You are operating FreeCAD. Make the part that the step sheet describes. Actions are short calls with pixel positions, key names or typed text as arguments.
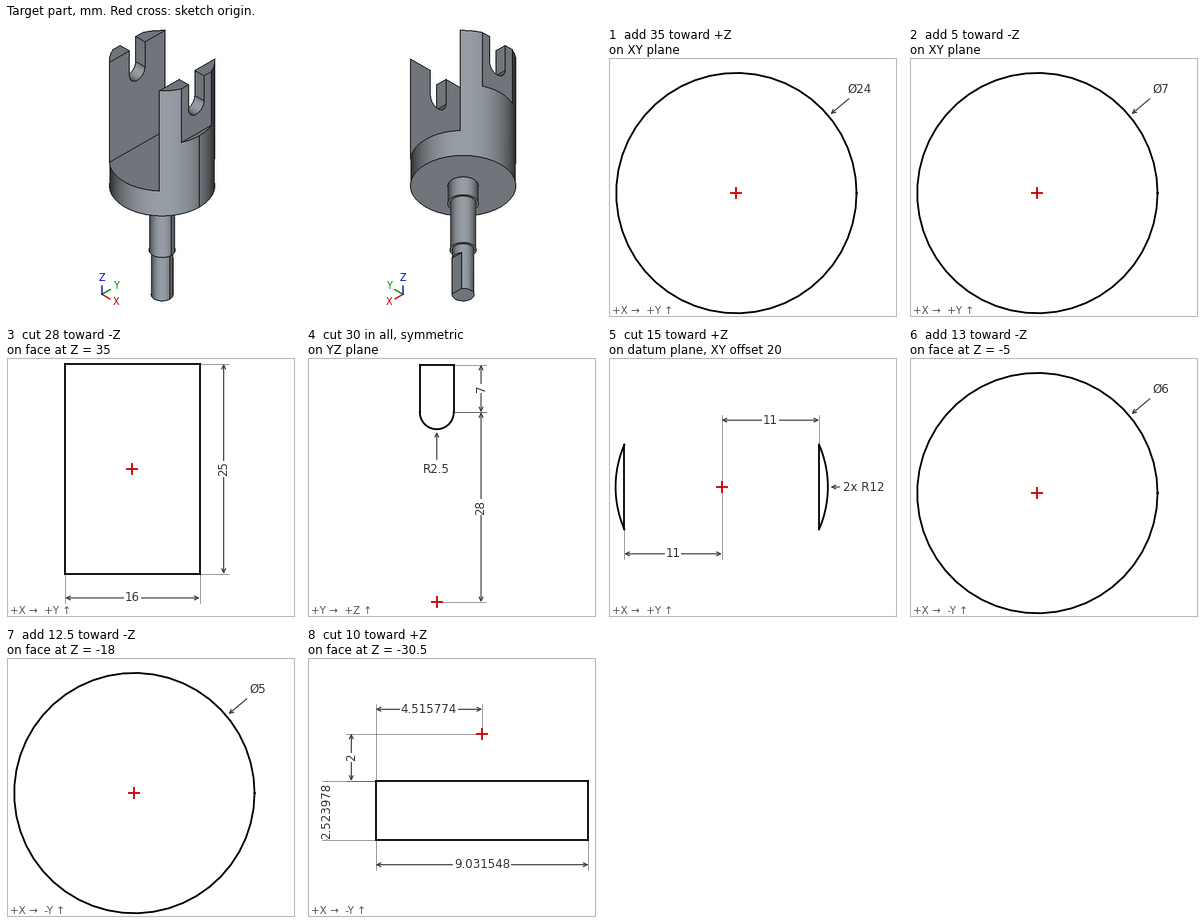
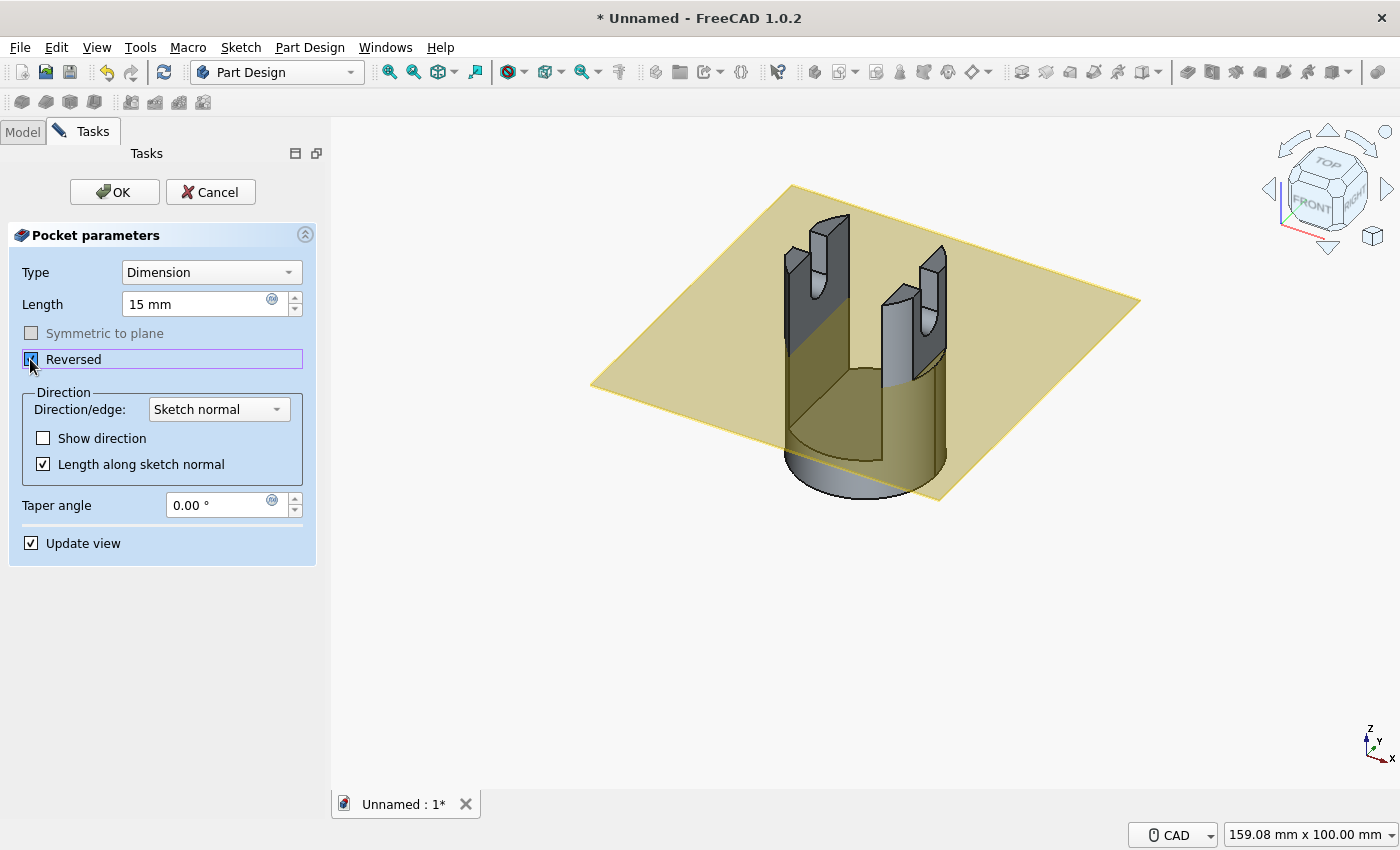
click(115, 192)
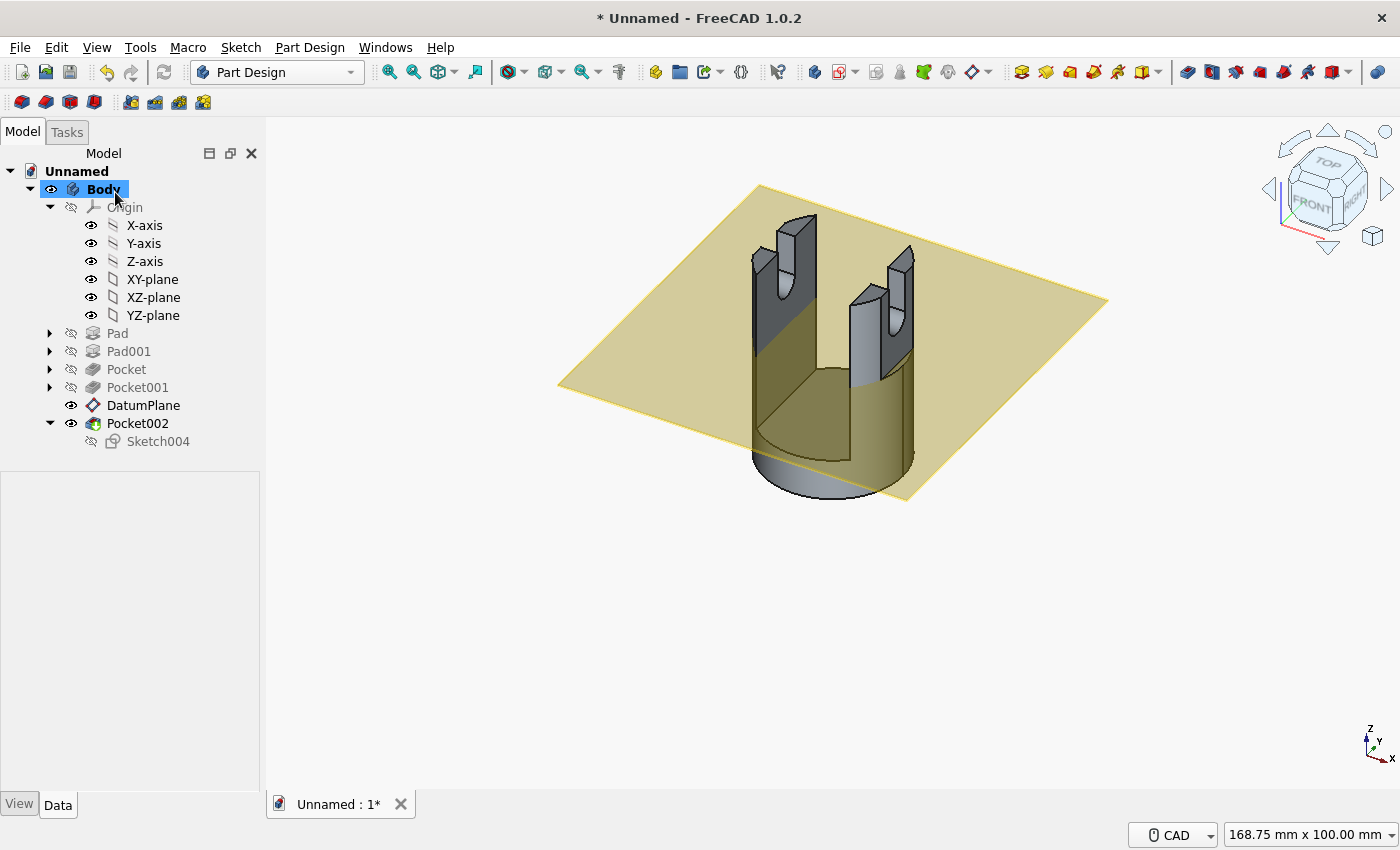
click(116, 405)
key(space)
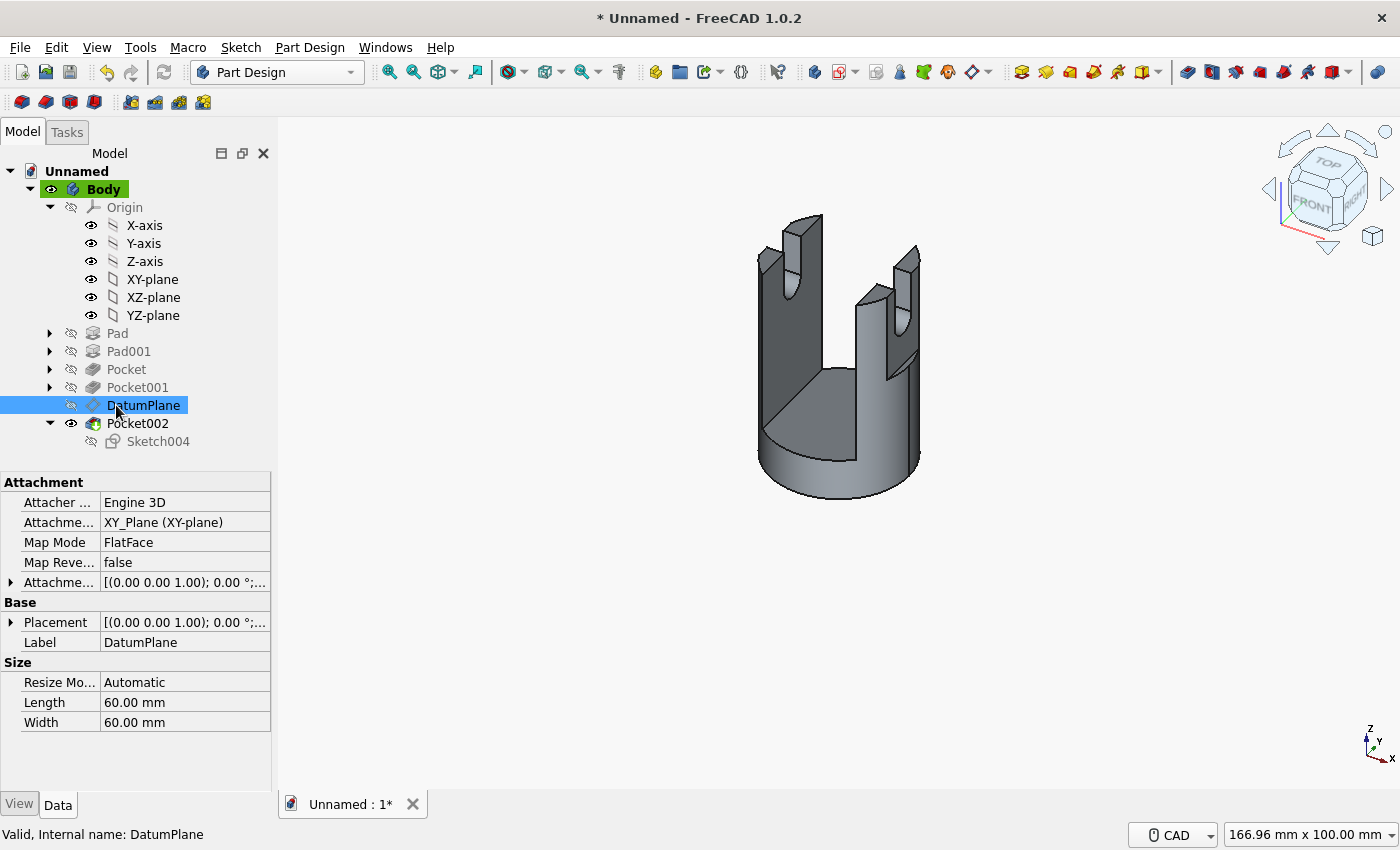
key(5)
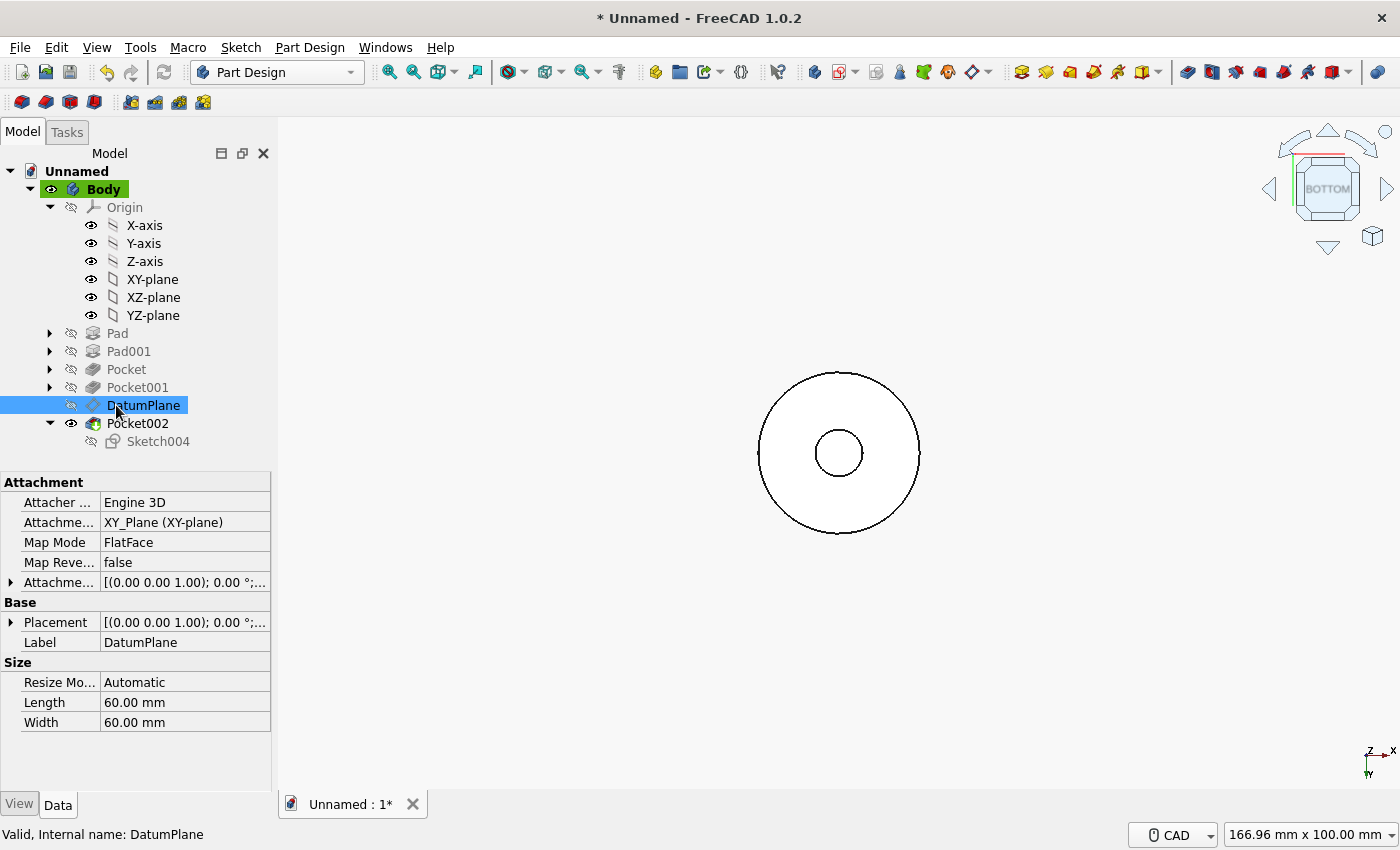
click(390, 72)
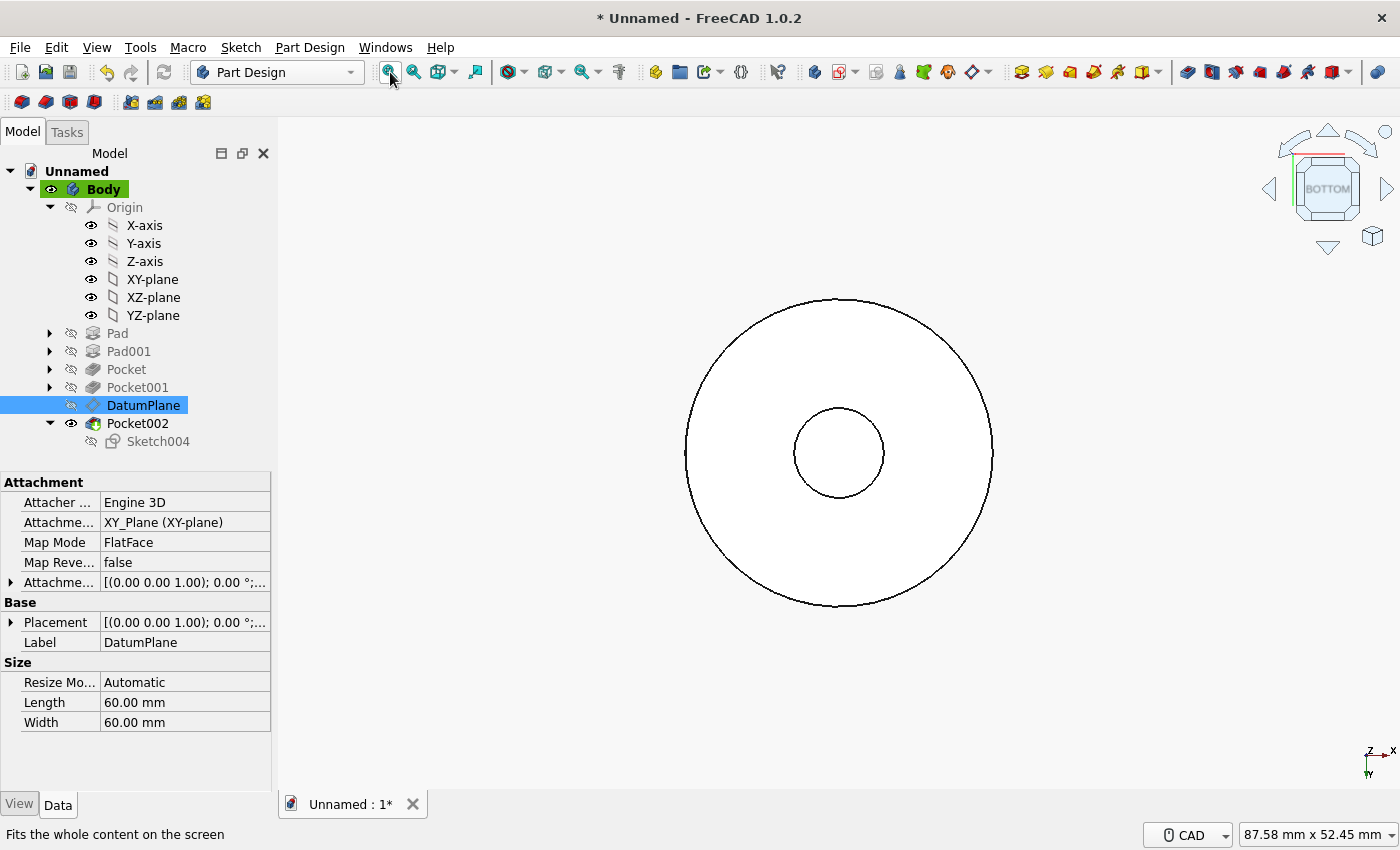
click(839, 452)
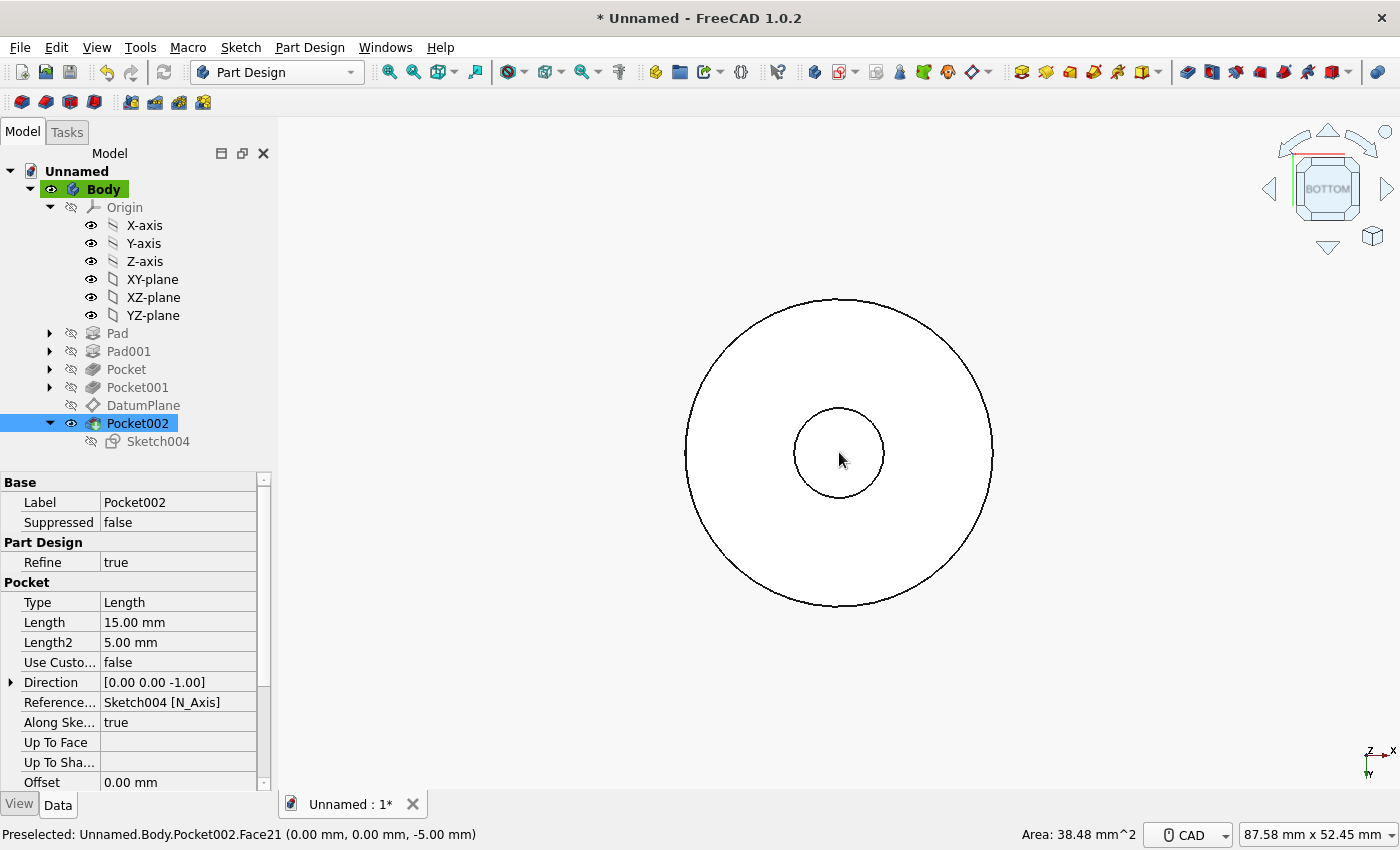
click(840, 72)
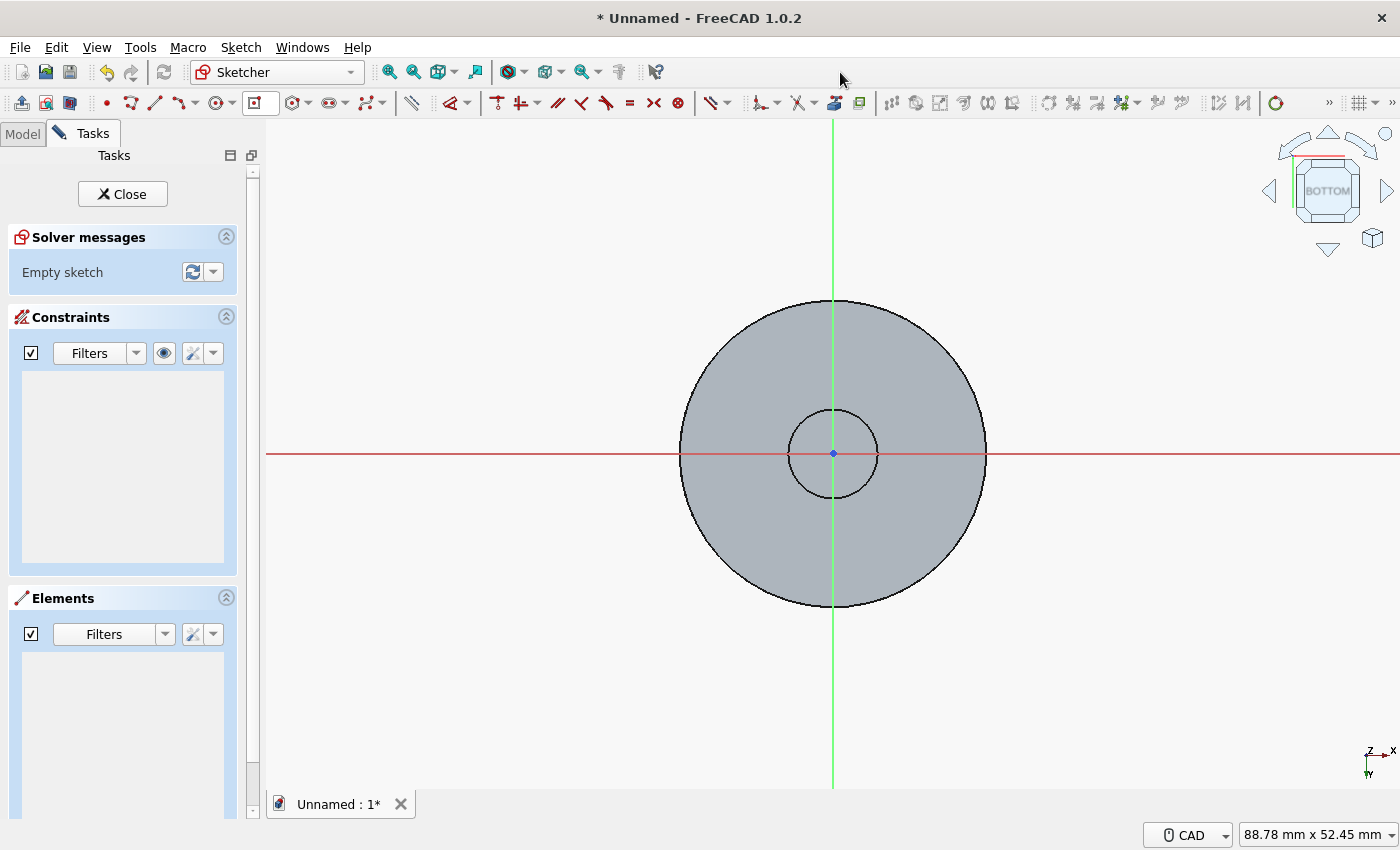
scroll(847, 454, up, 9)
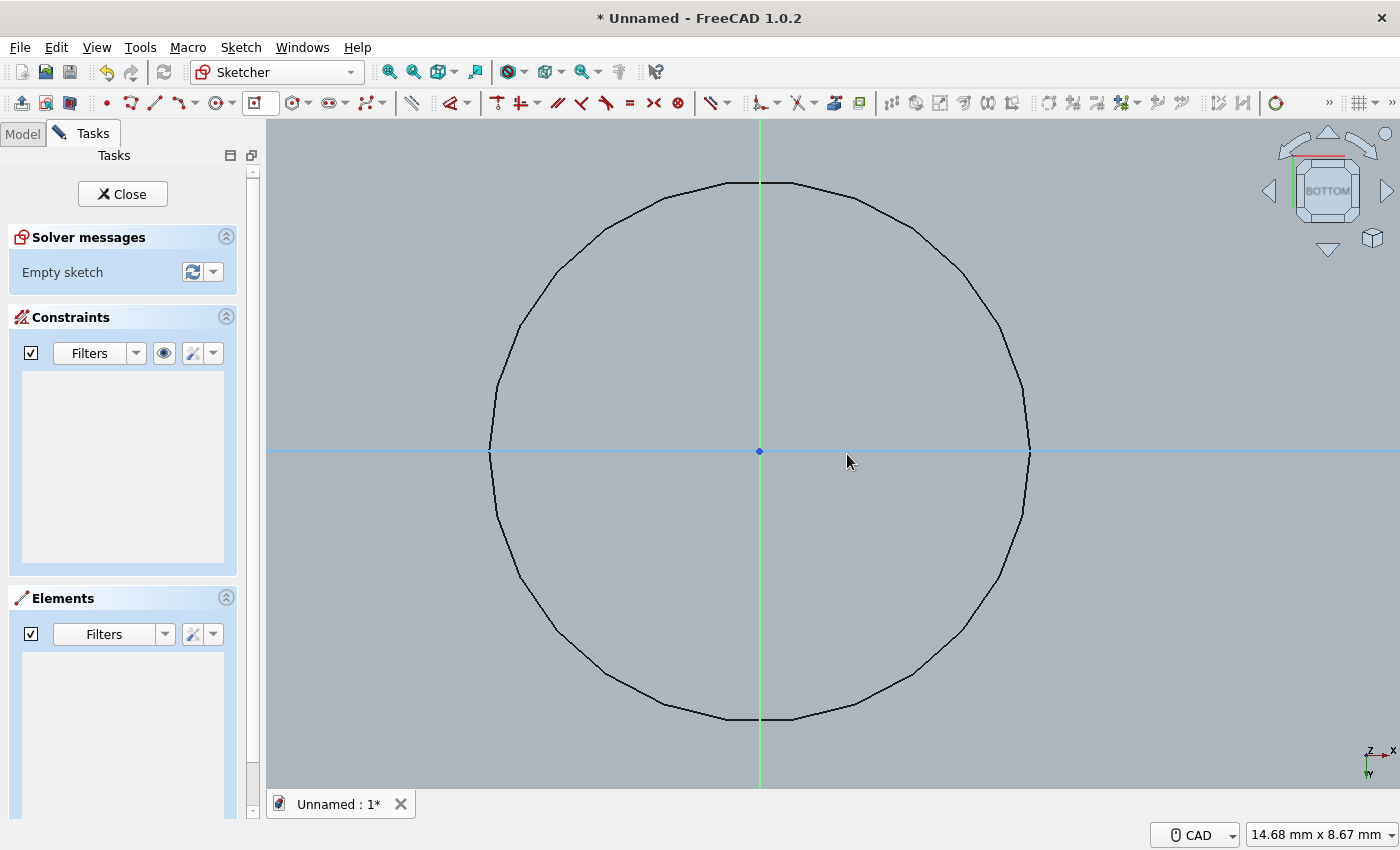
key(g)
key(c)